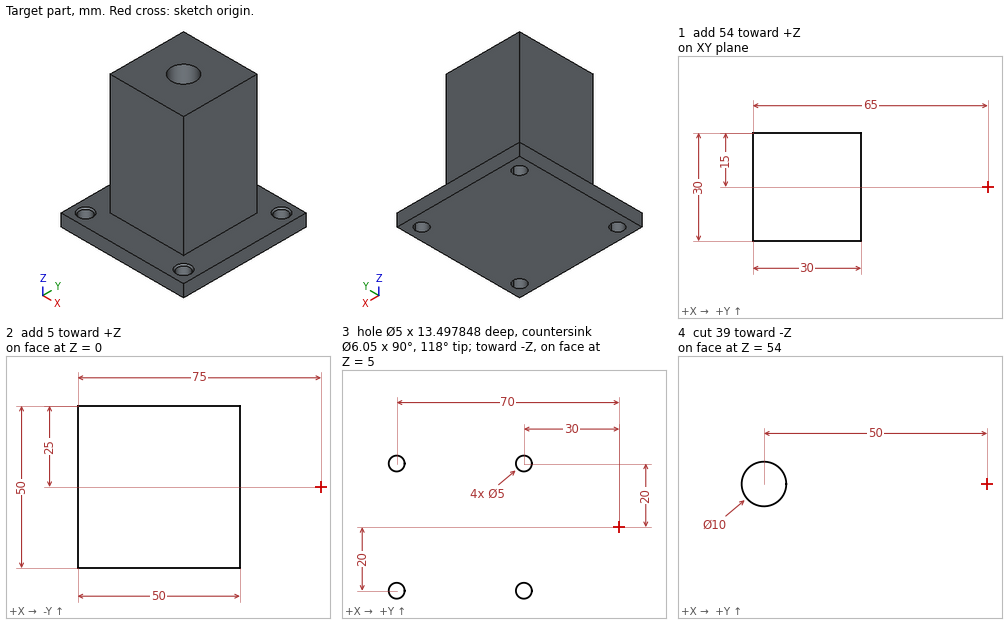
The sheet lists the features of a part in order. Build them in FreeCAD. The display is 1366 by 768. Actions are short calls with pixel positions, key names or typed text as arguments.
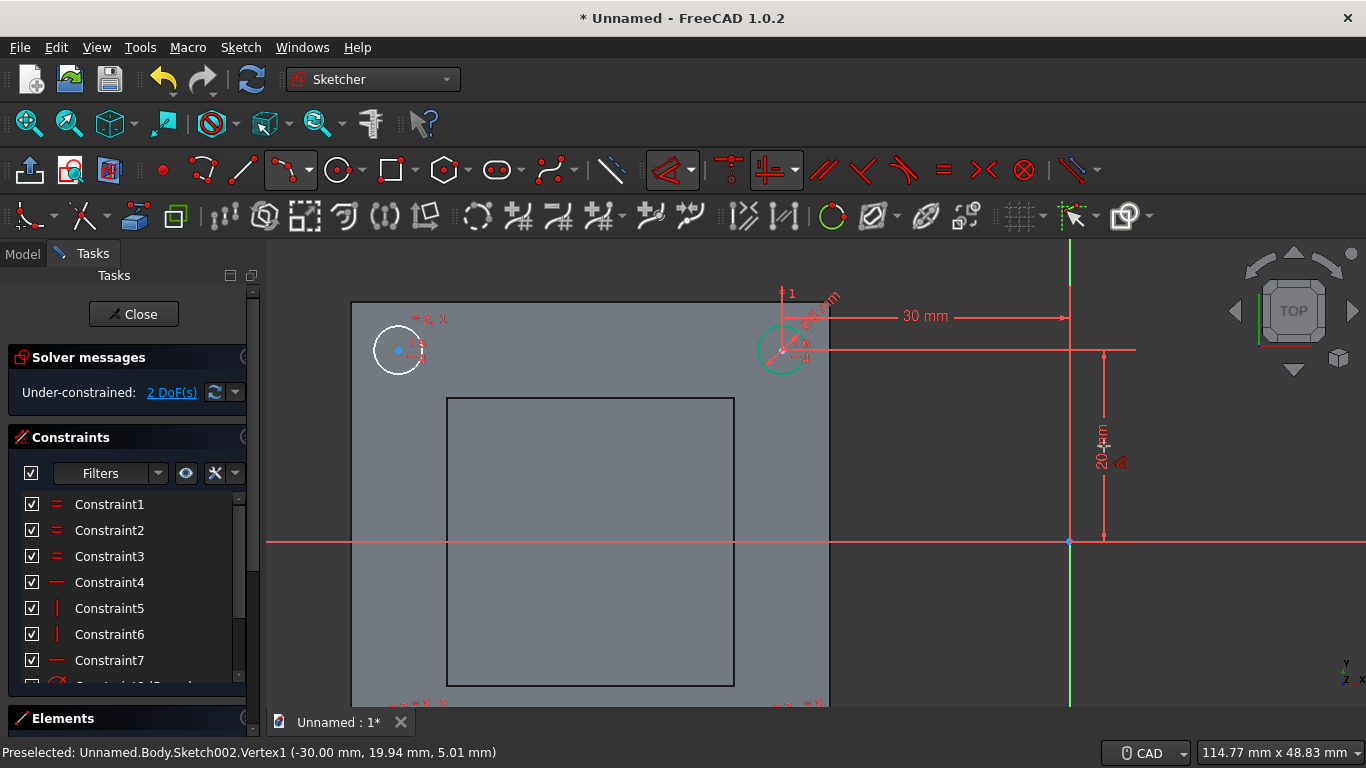
click(398, 350)
click(734, 316)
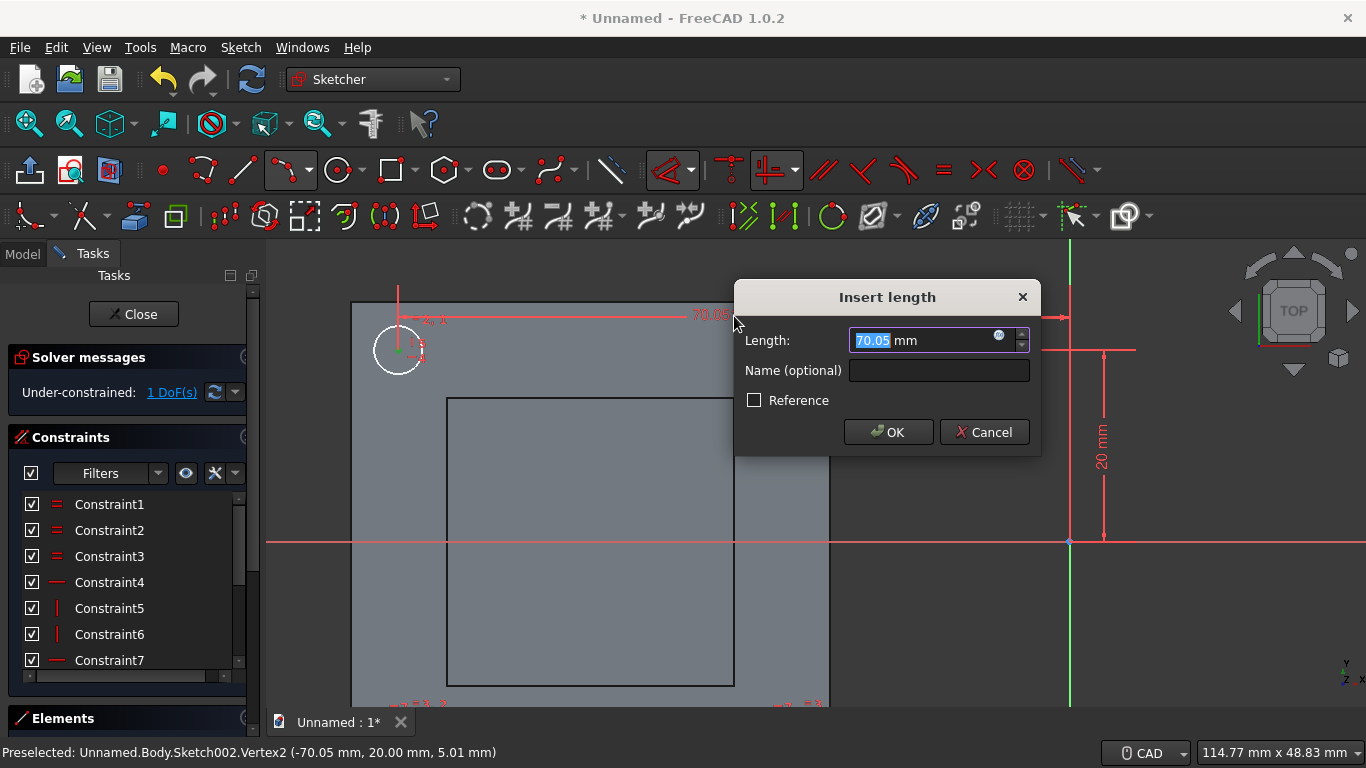
text(70)
key(Return)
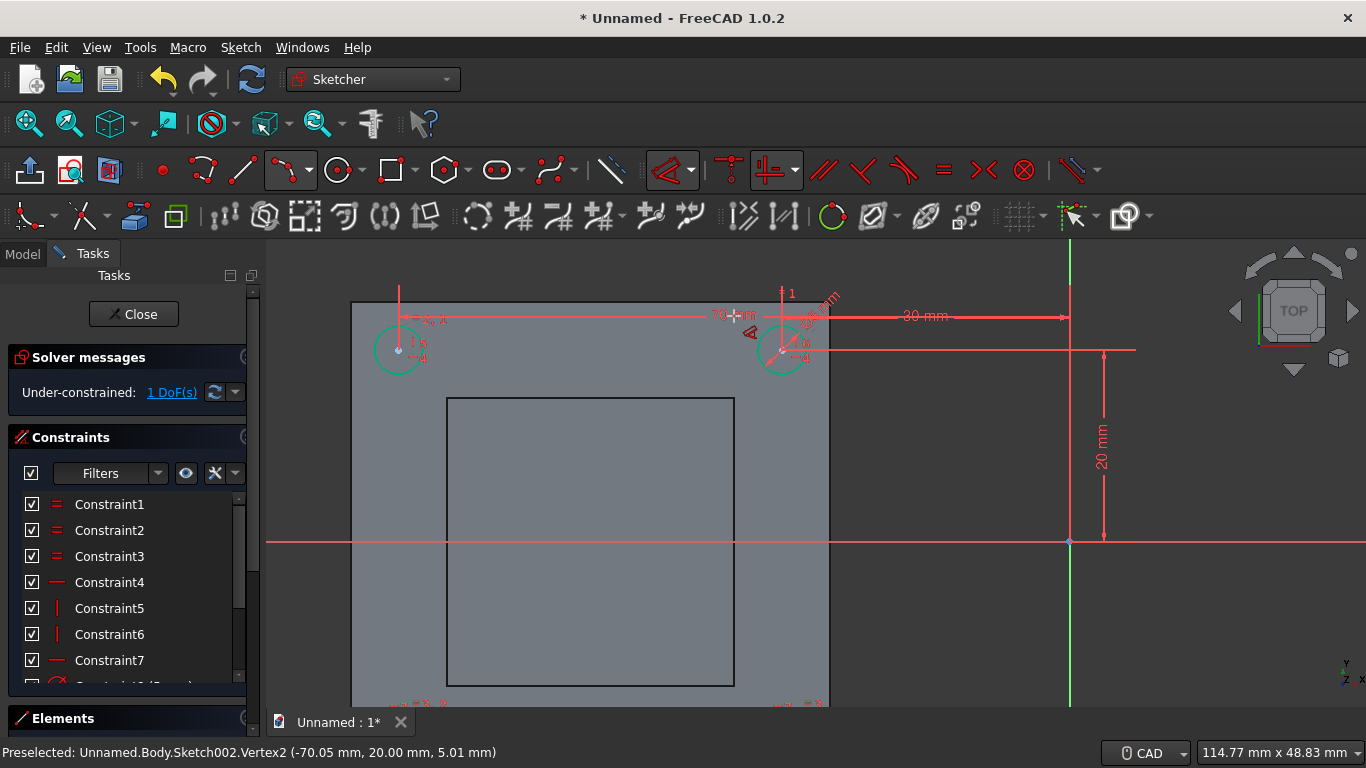
scroll(799, 333, down, 2)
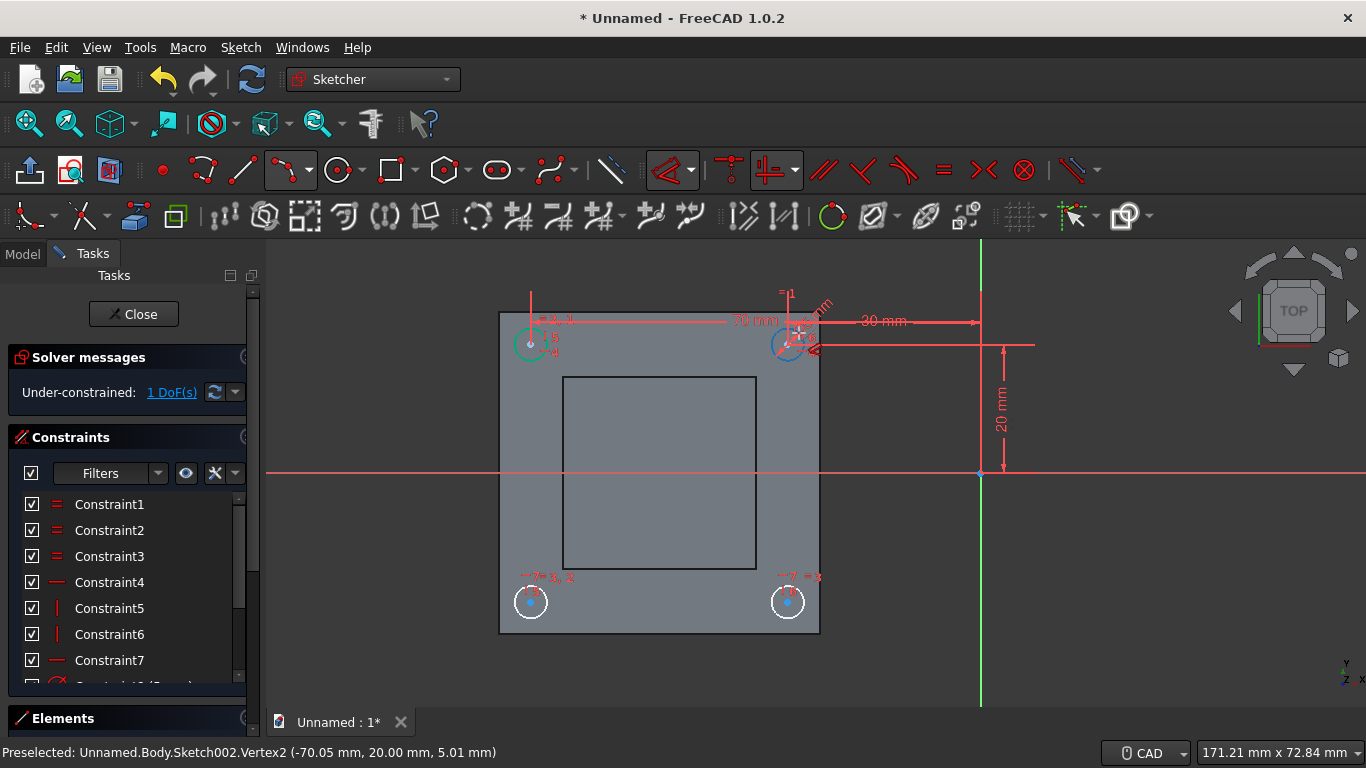
click(531, 602)
click(1015, 538)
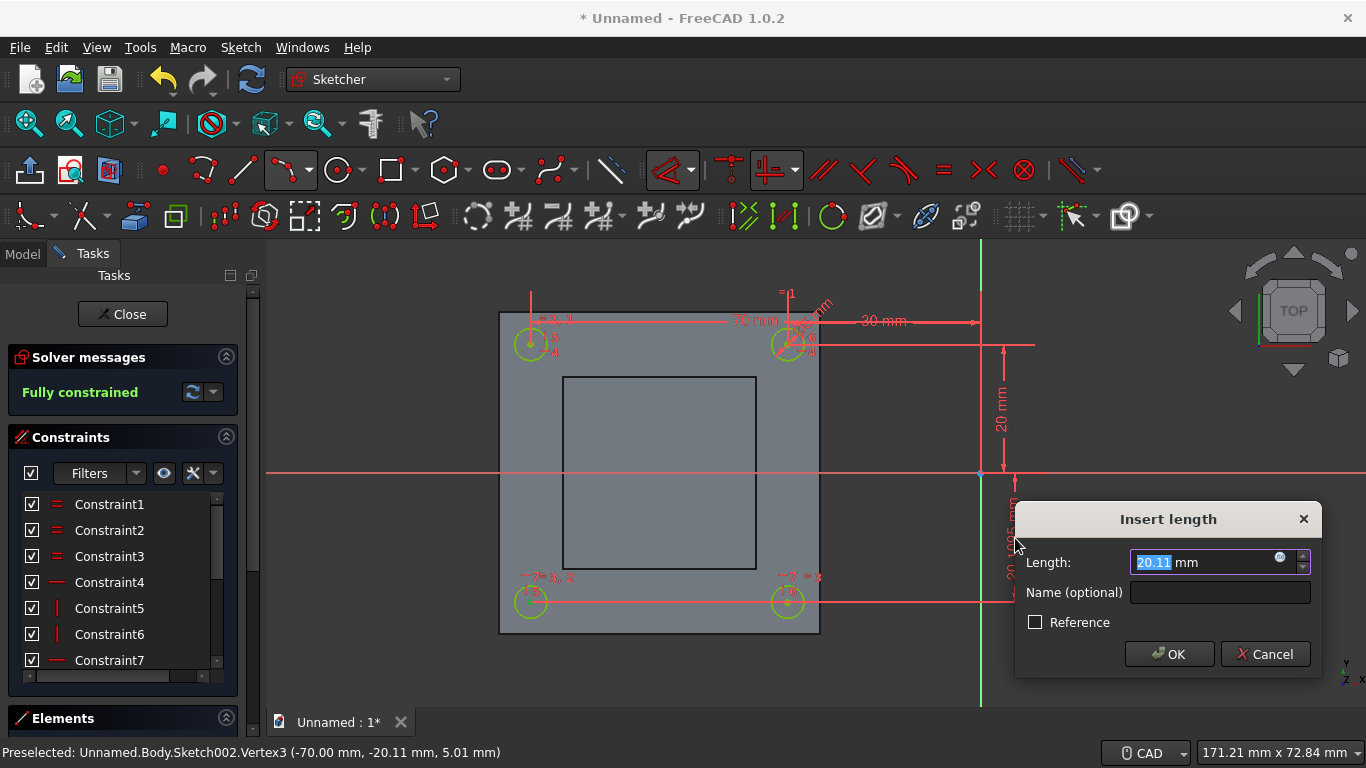
text(20)
key(Return)
key(Escape)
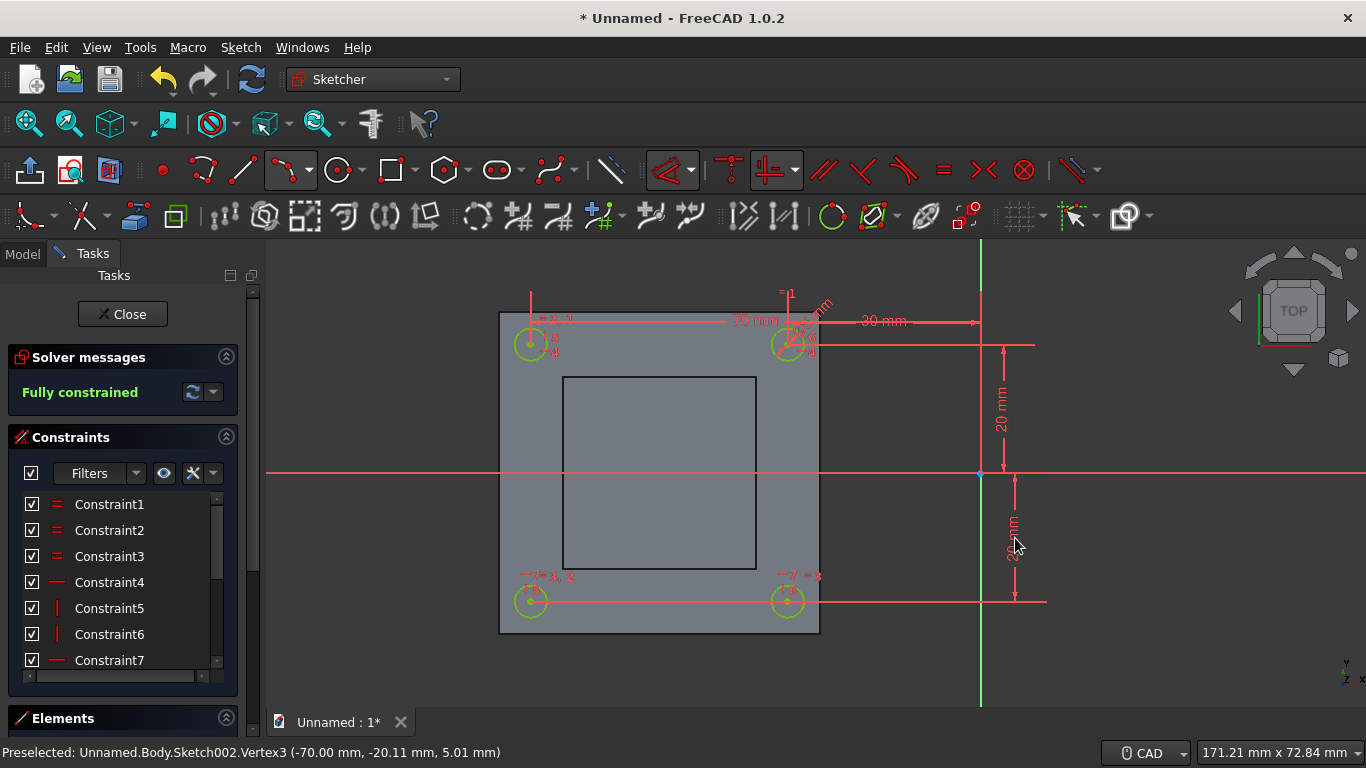
click(123, 314)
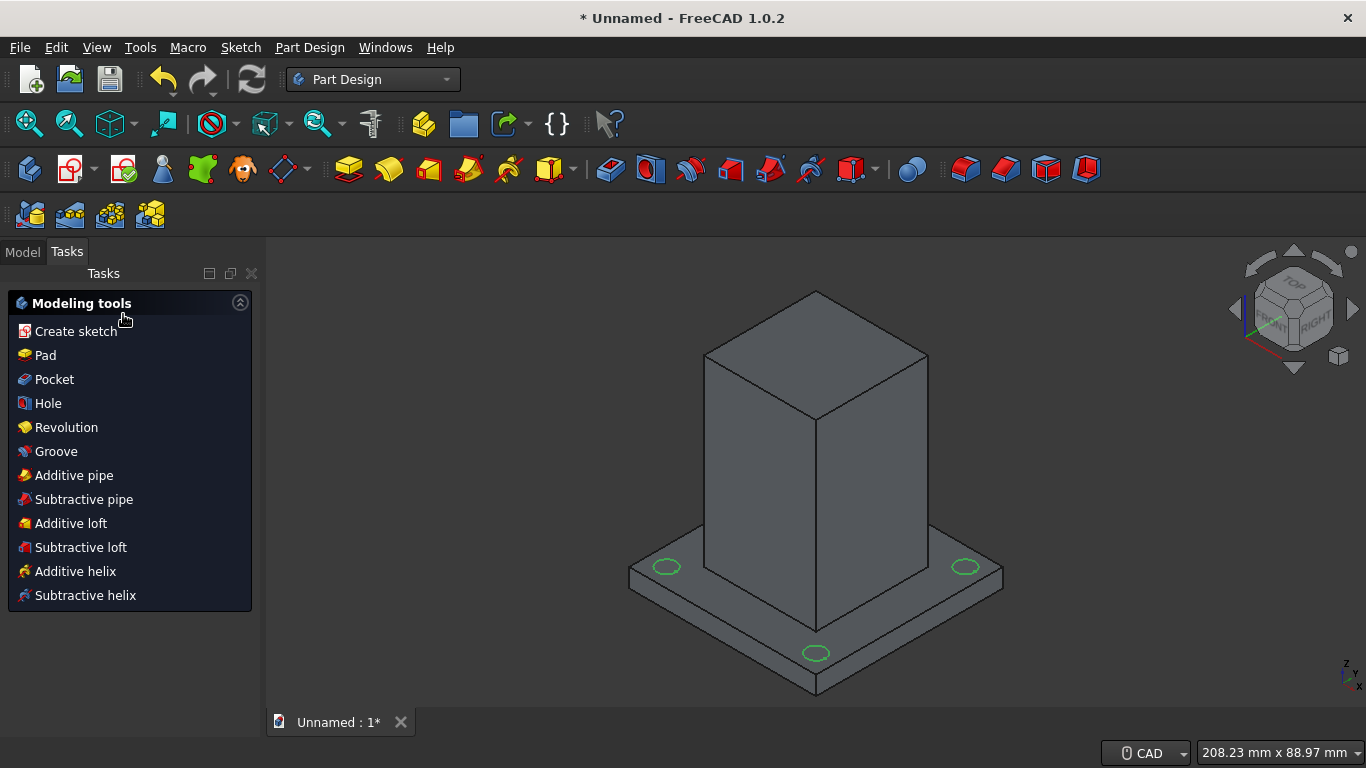
click(652, 170)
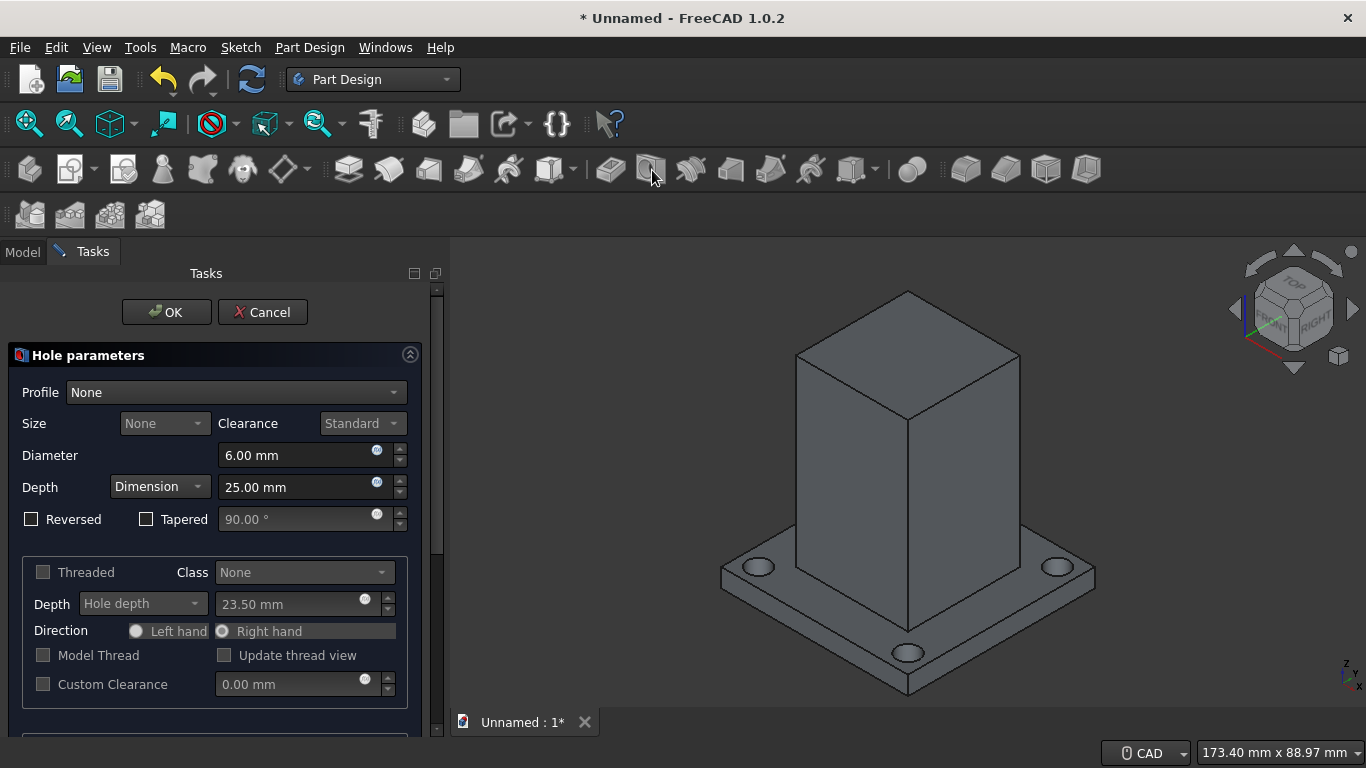
triple_click(305, 455)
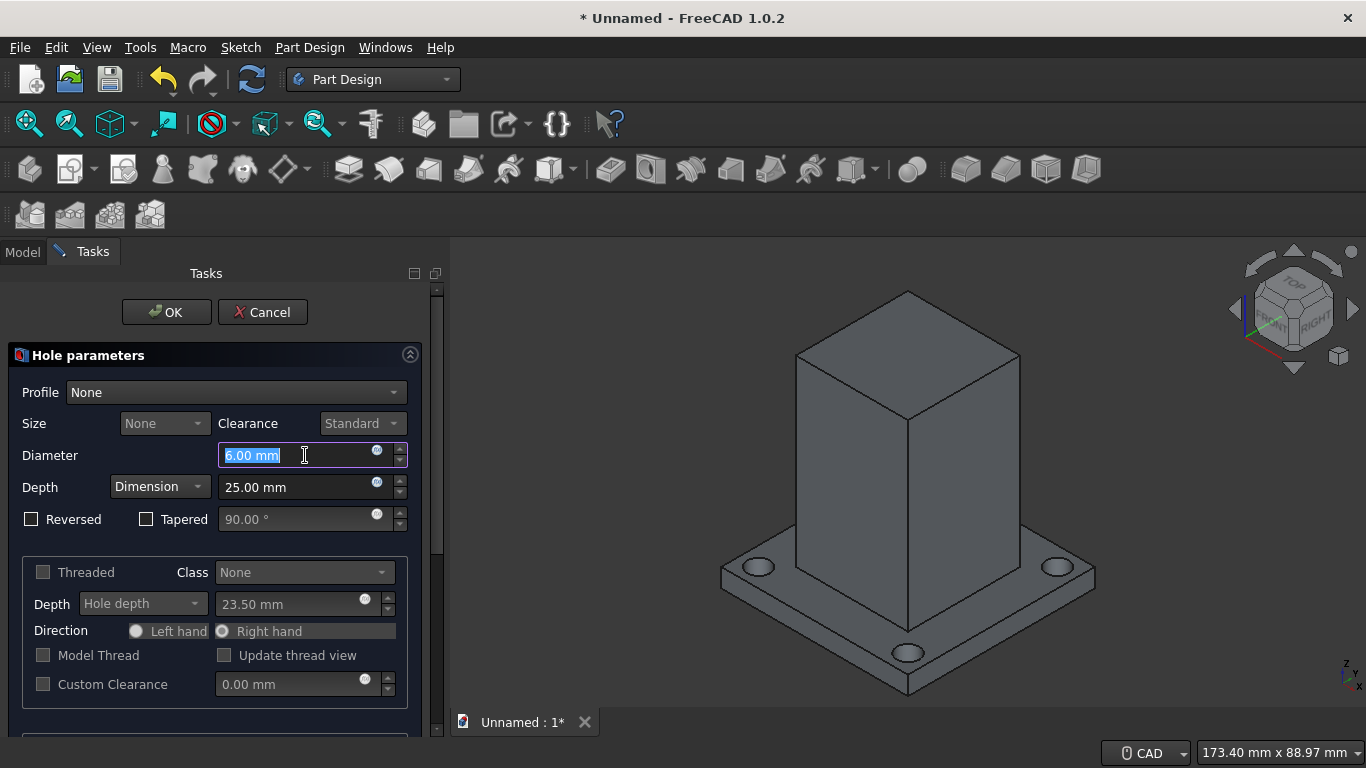
text(5)
key(Tab)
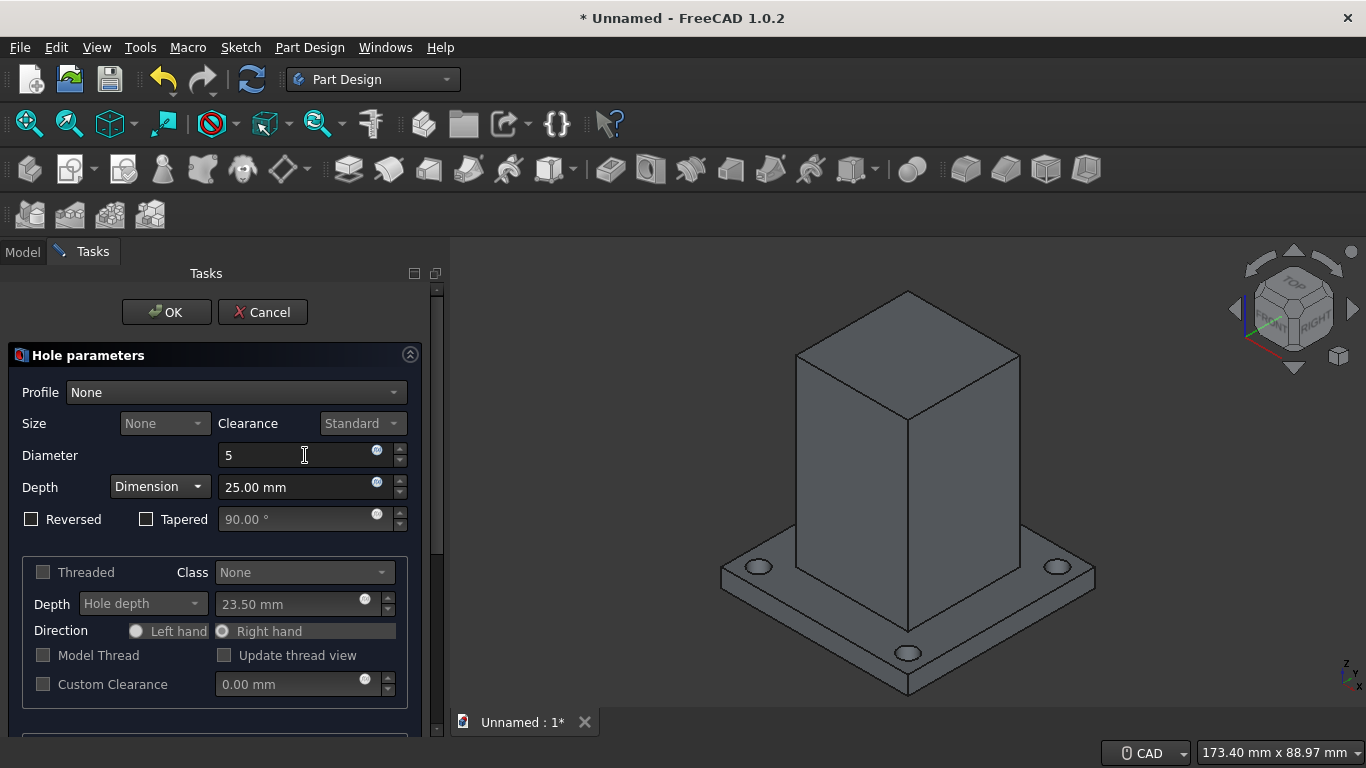
triple_click(305, 487)